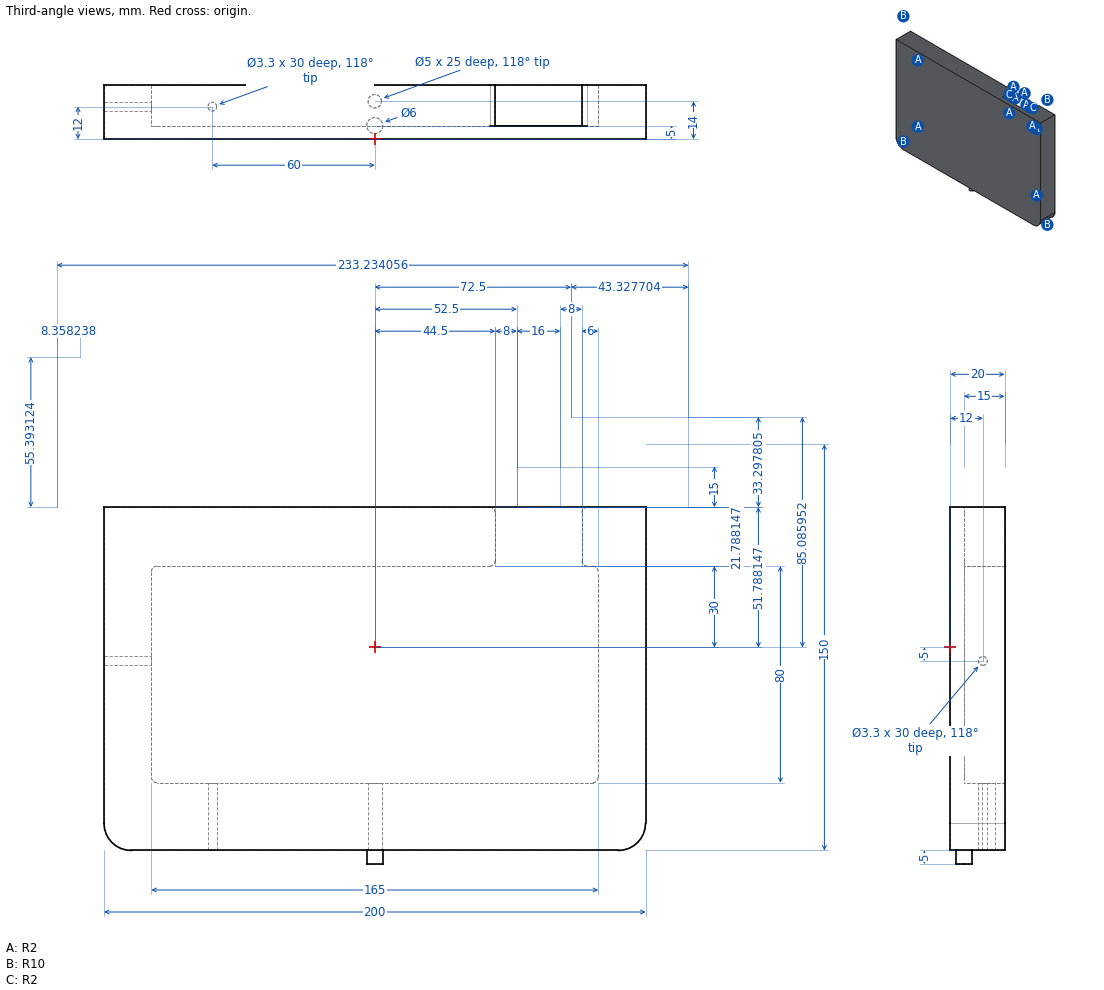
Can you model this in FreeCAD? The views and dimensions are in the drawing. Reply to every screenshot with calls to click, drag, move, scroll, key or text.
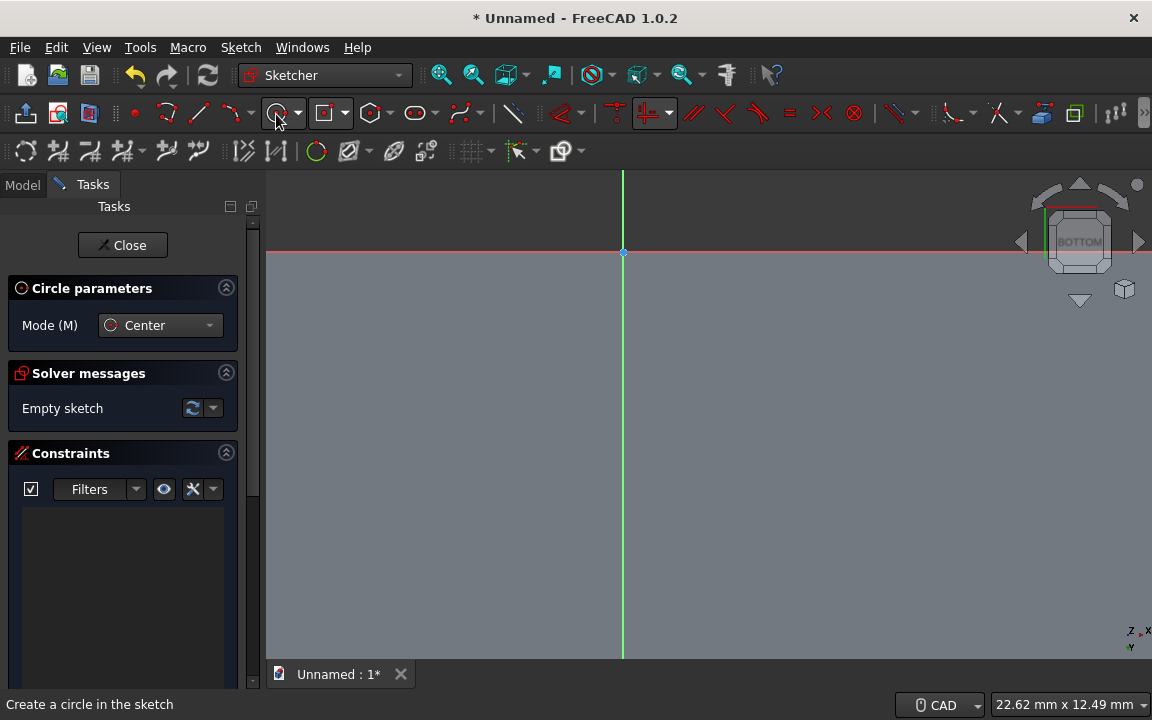
click(623, 448)
click(706, 365)
key(Escape)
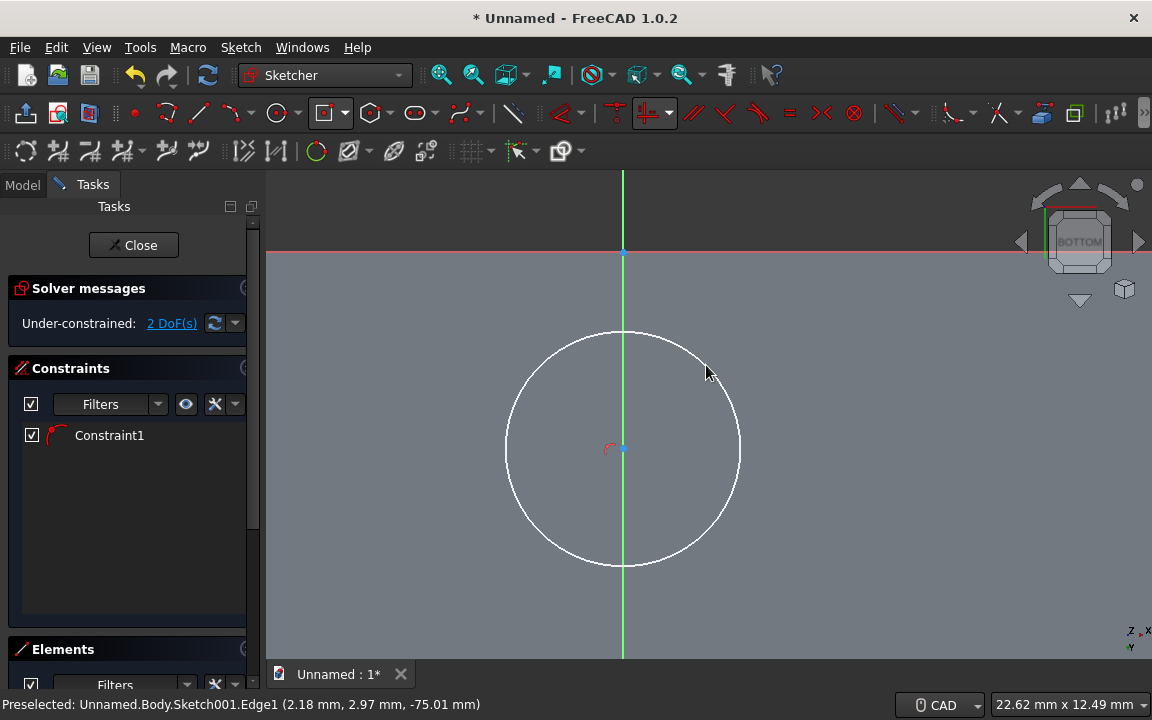
key(d)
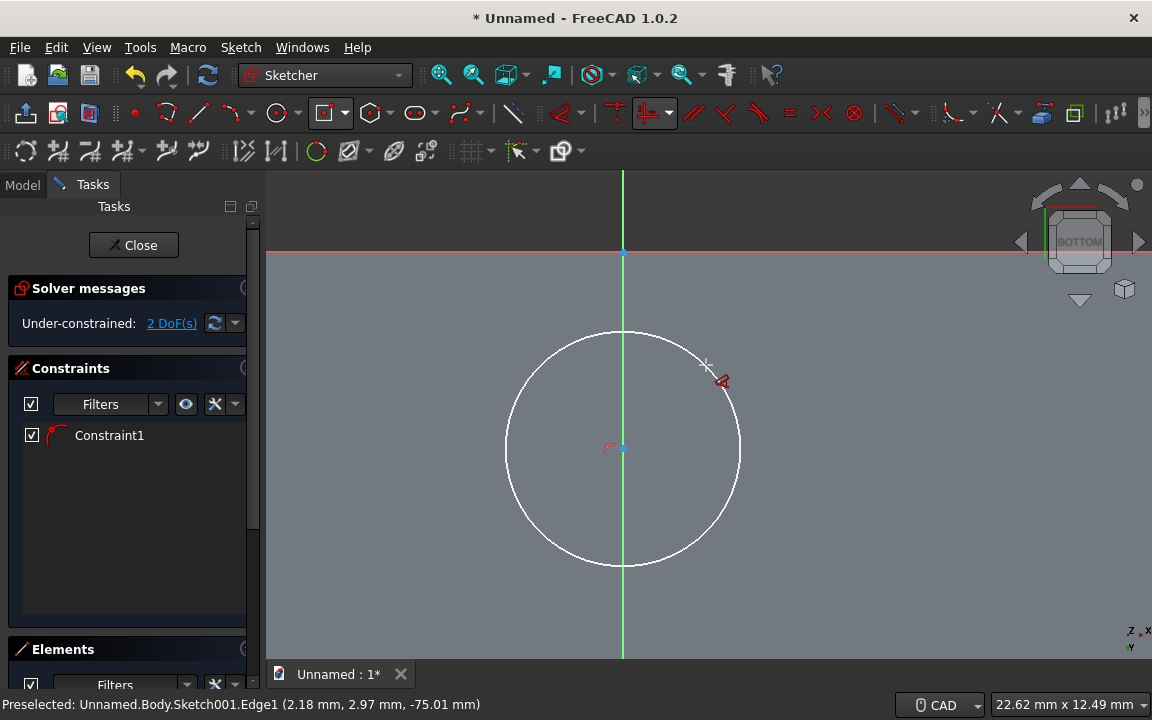
click(706, 366)
click(729, 343)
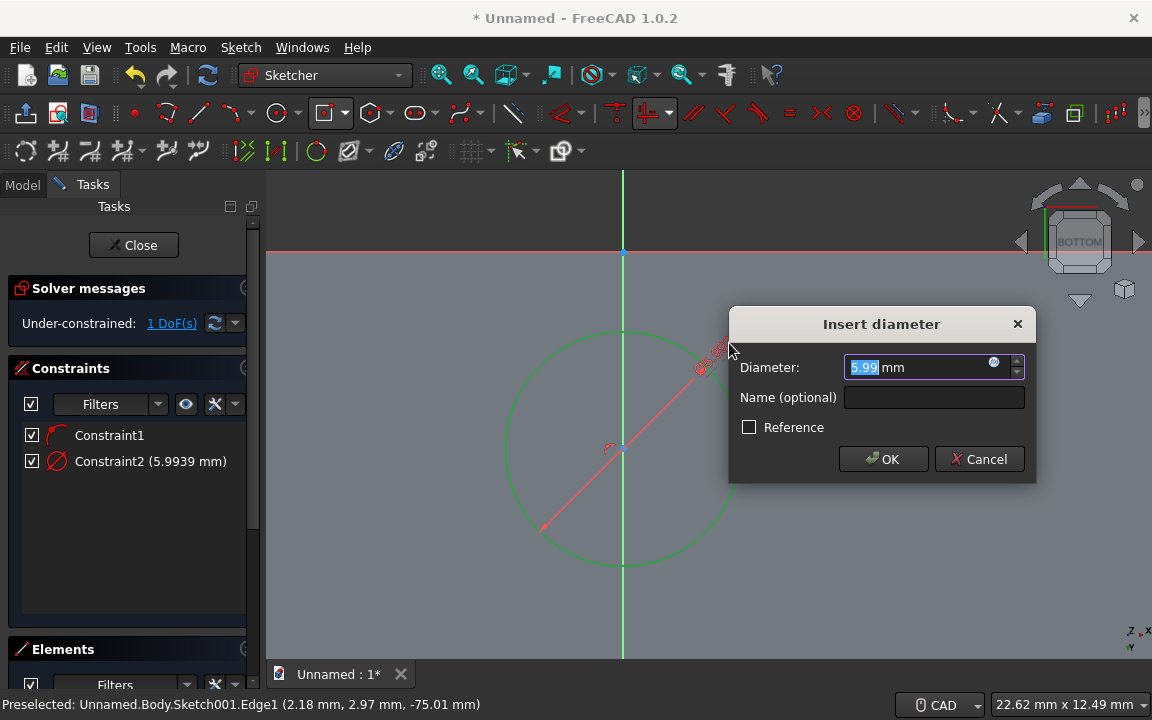
text(6)
key(Return)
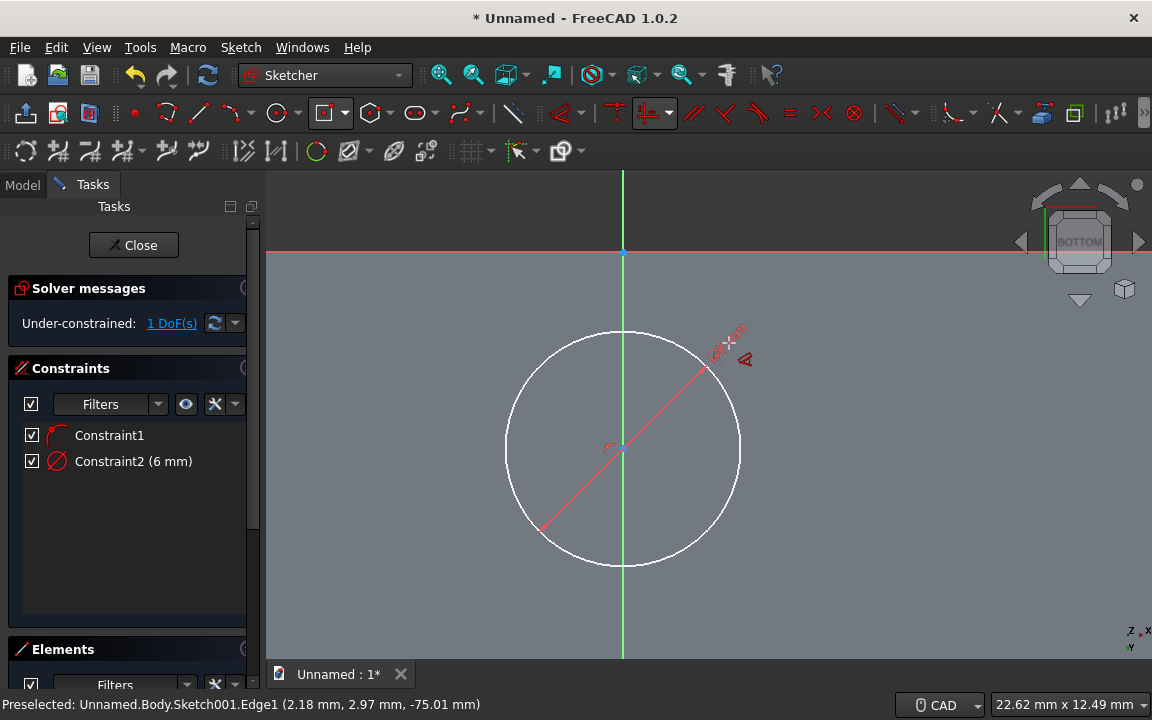
click(623, 449)
click(657, 351)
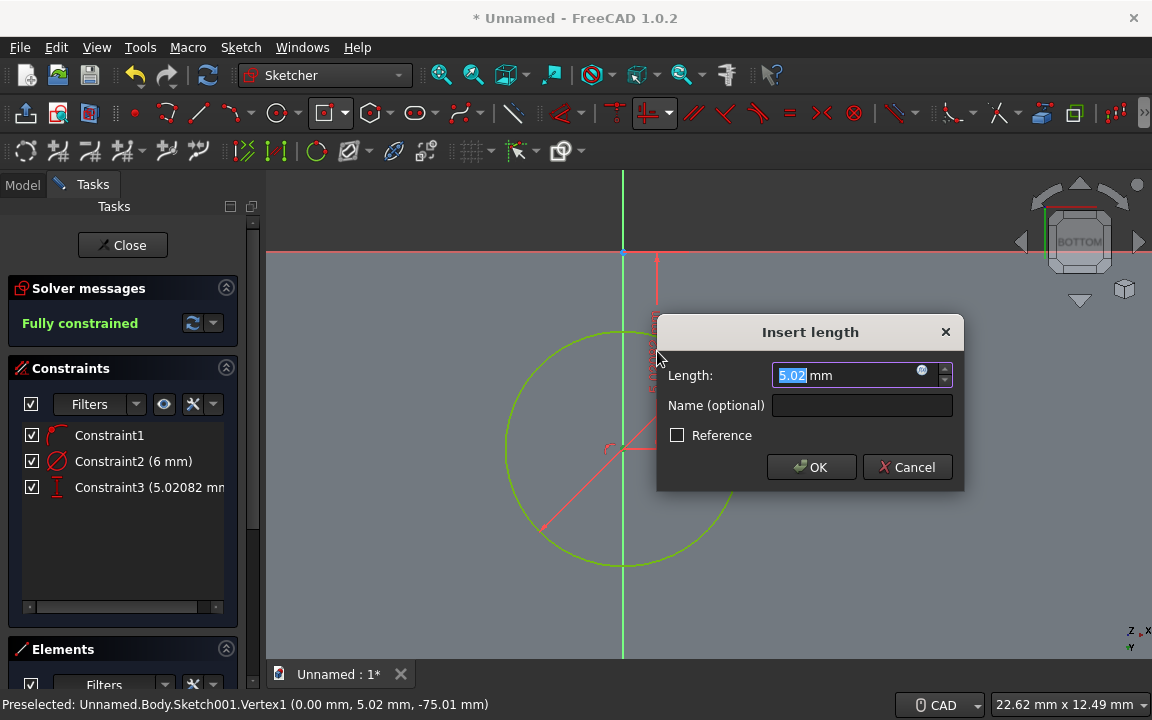
text(5)
key(Return)
key(Escape)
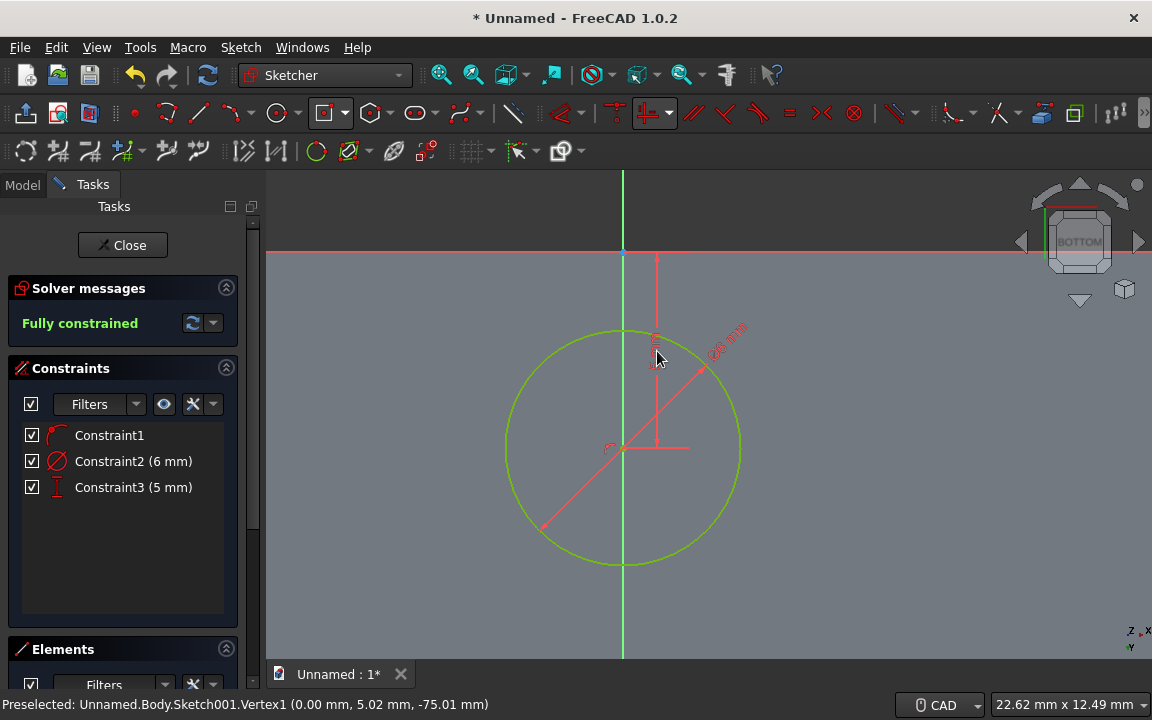
click(123, 245)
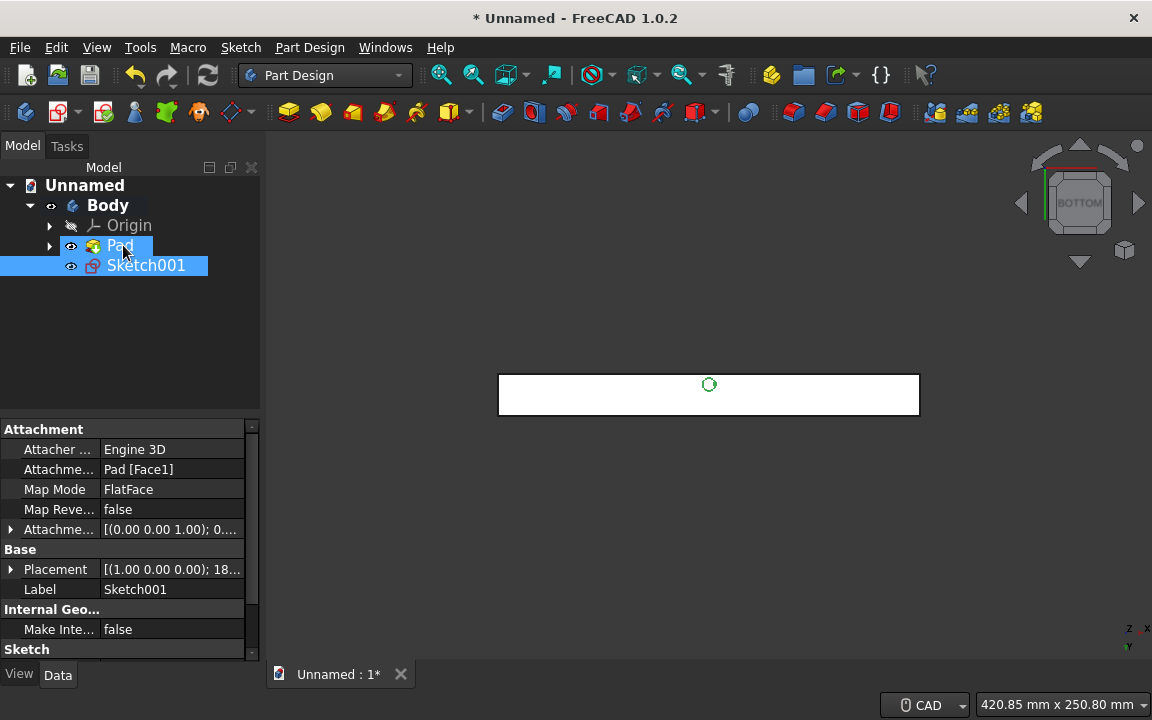
click(290, 112)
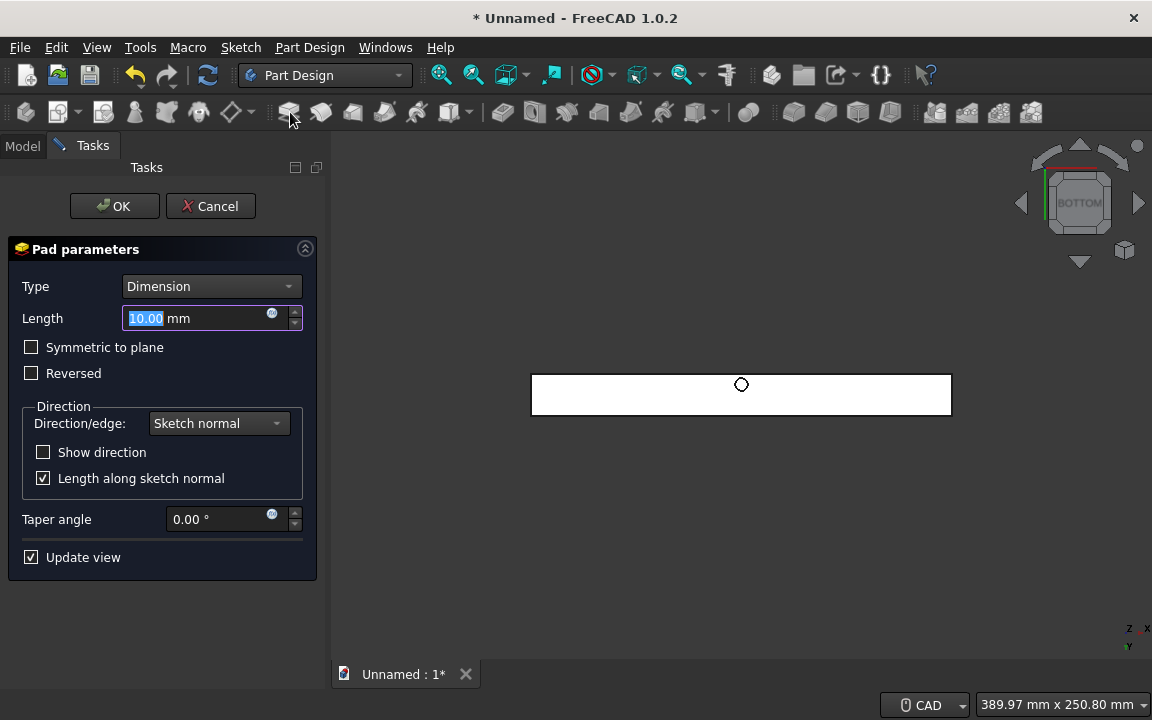
text(5)
key(Tab)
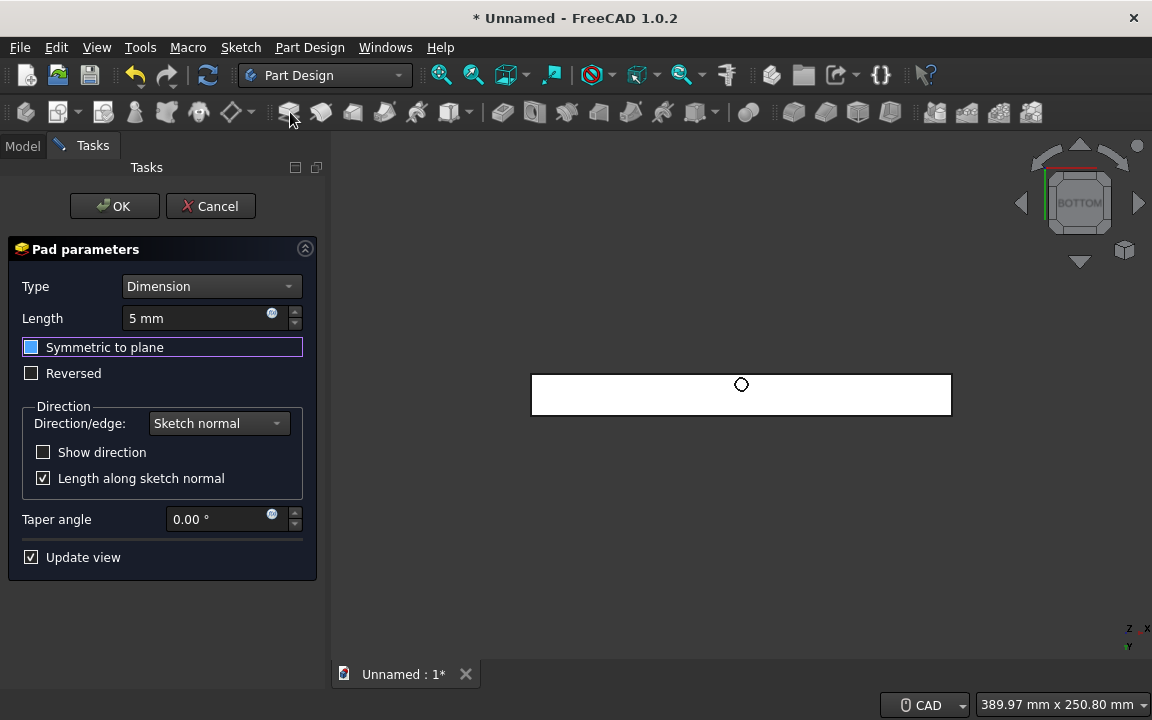
click(115, 206)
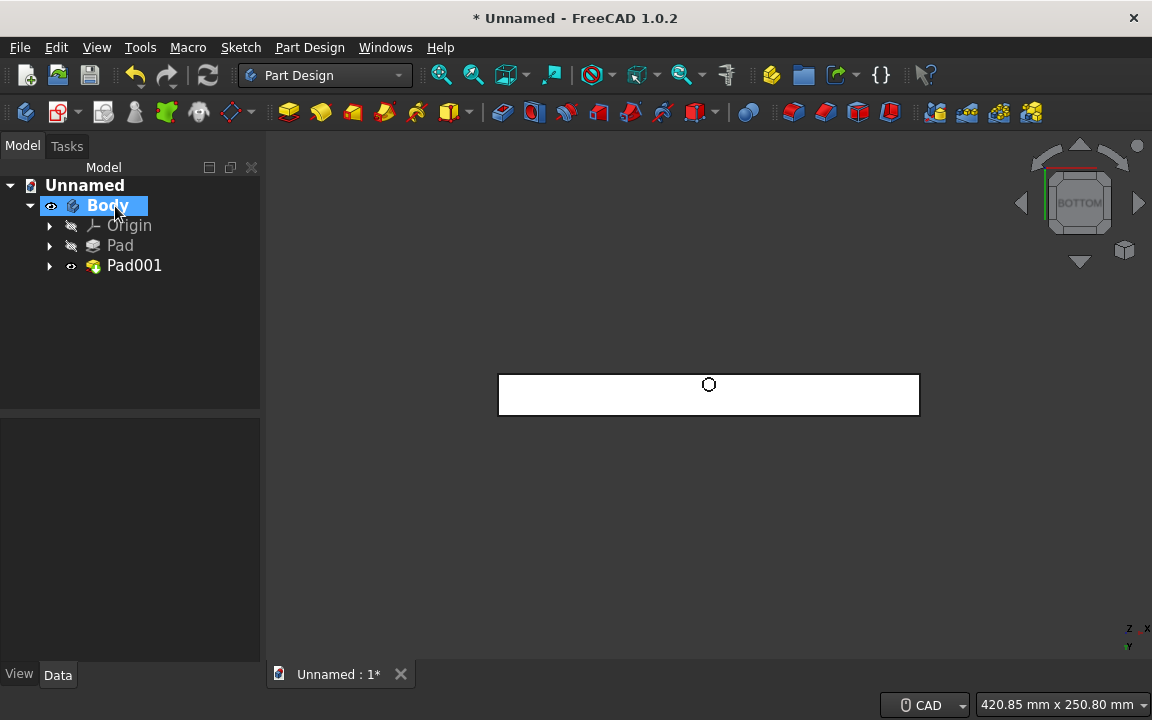
click(889, 394)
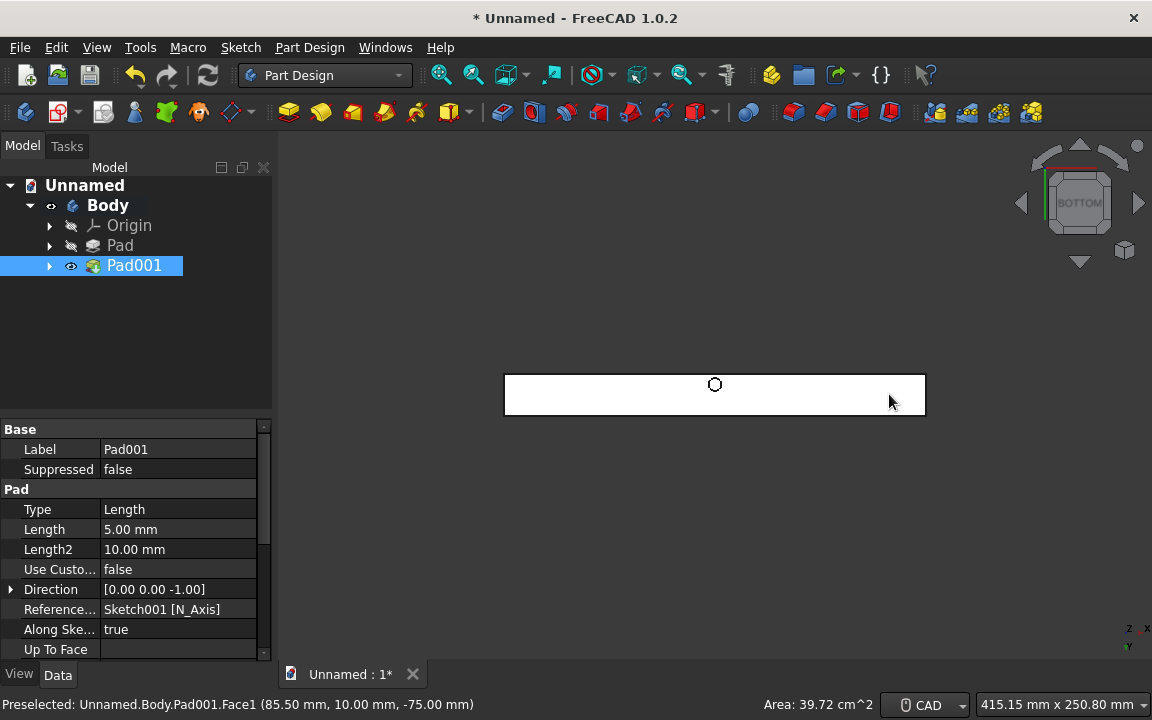
click(58, 112)